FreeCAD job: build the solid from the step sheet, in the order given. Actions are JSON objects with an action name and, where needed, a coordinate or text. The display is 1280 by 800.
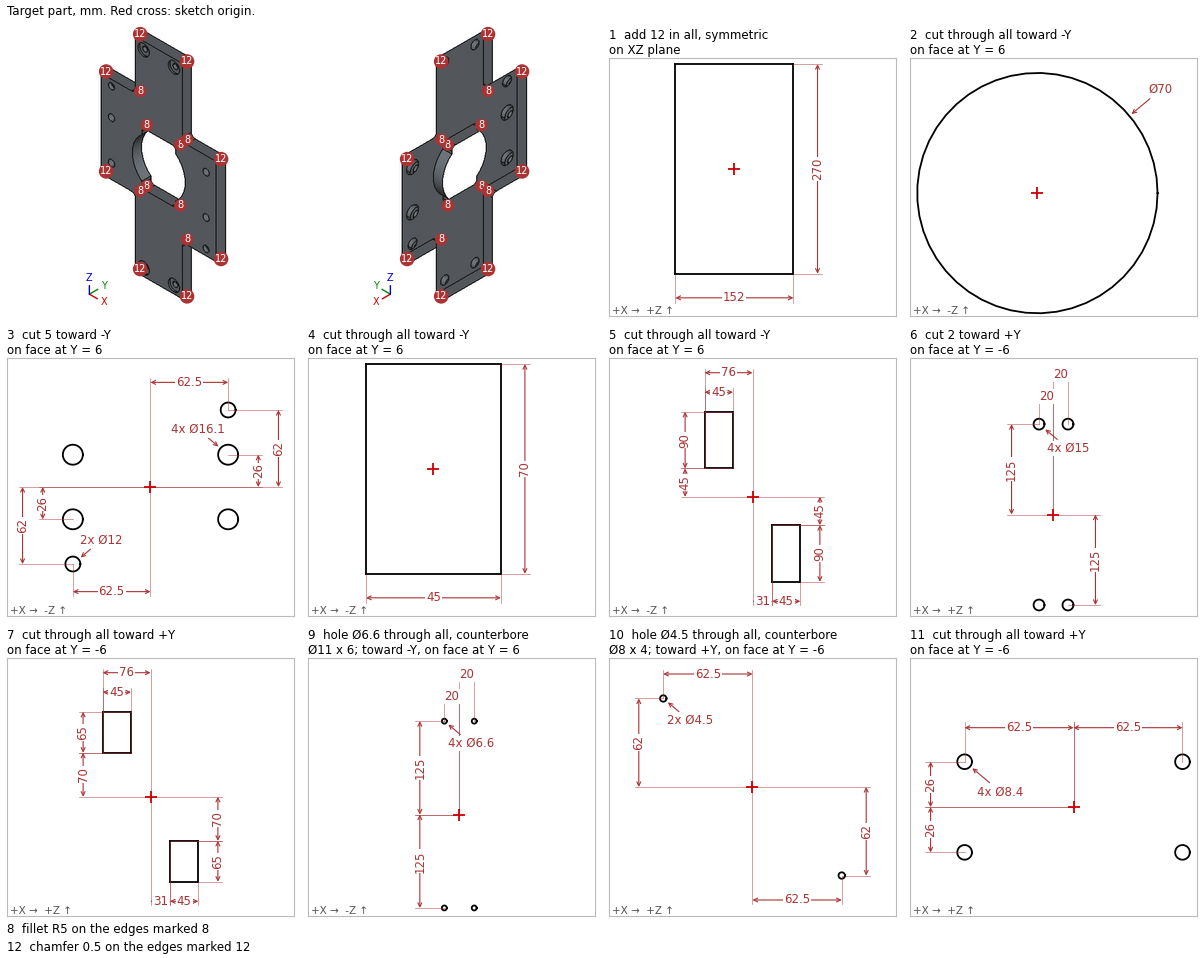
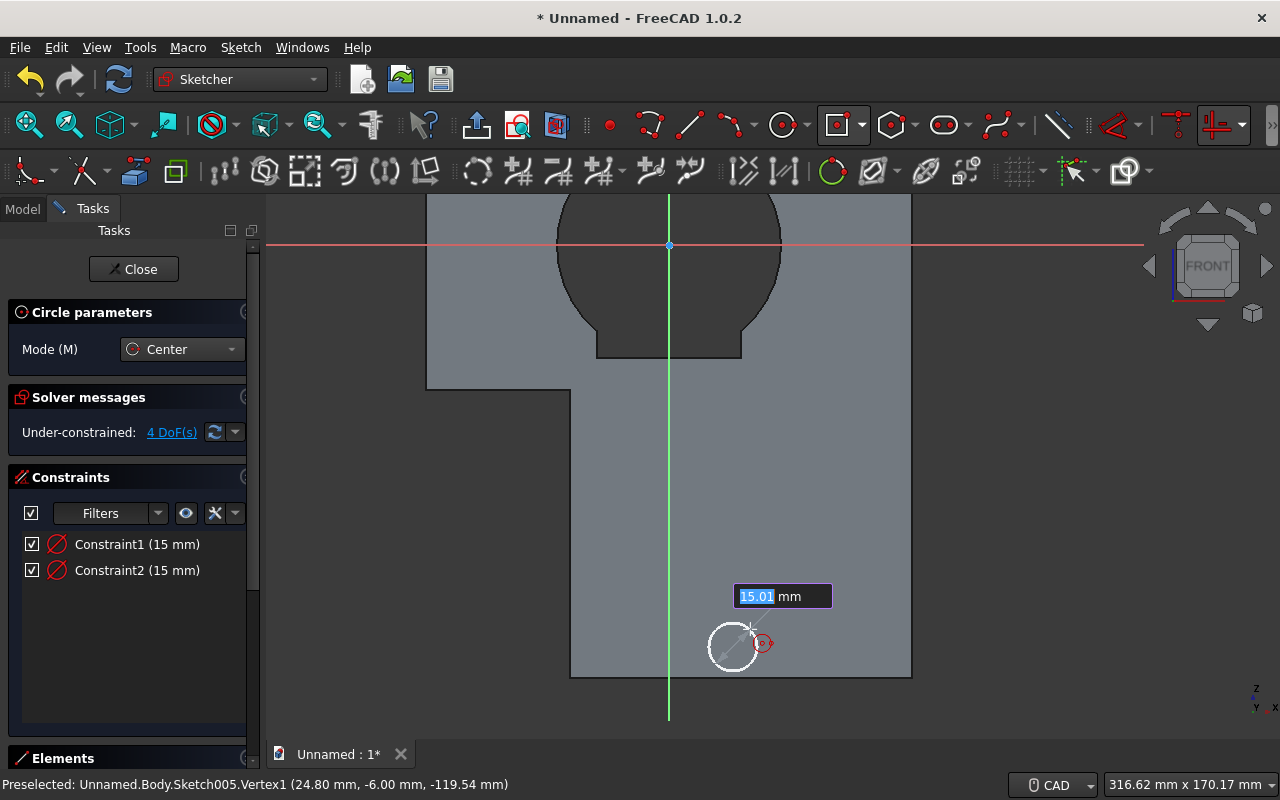
{"action": "type", "text": "15"}
{"action": "key", "text": "Return"}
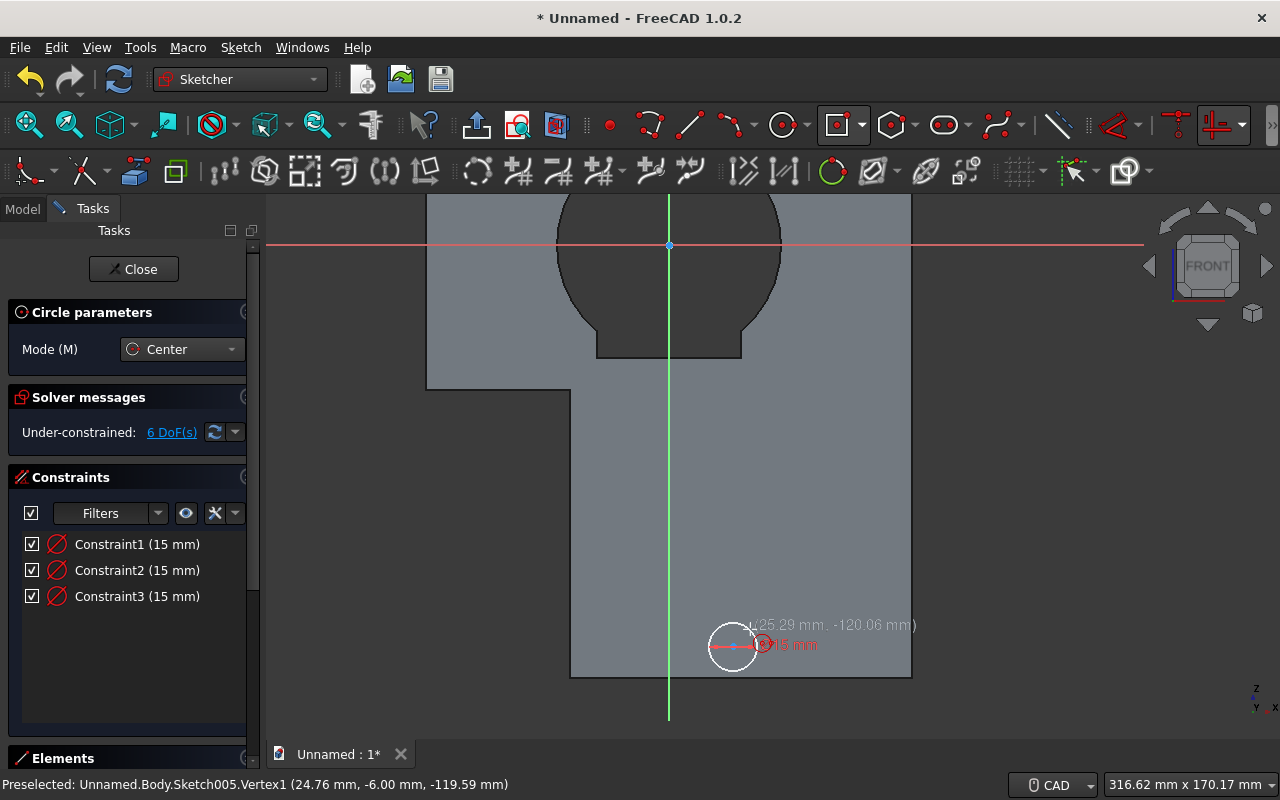
{"action": "left_click", "coordinate": [605, 646]}
{"action": "mouse_move", "coordinate": [622, 629]}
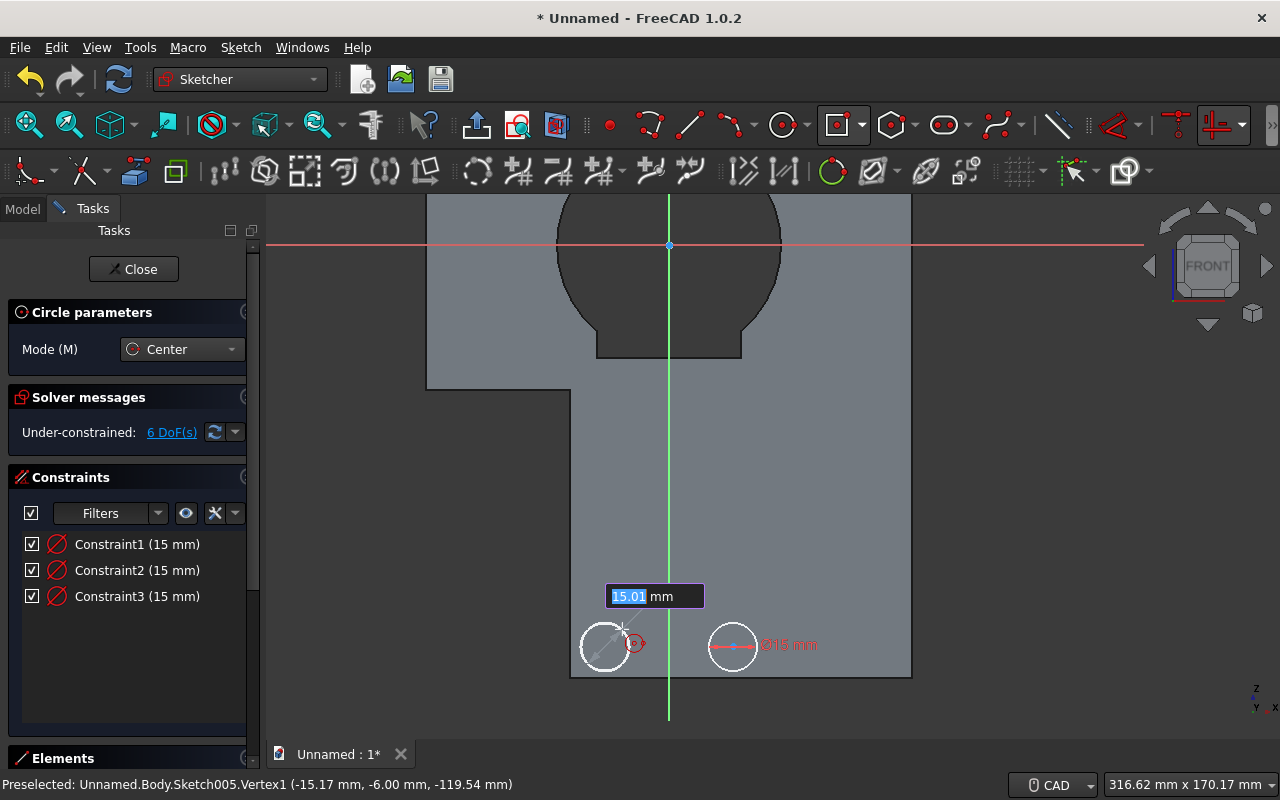
{"action": "type", "text": "15"}
{"action": "key", "text": "Return"}
{"action": "key", "text": "Escape"}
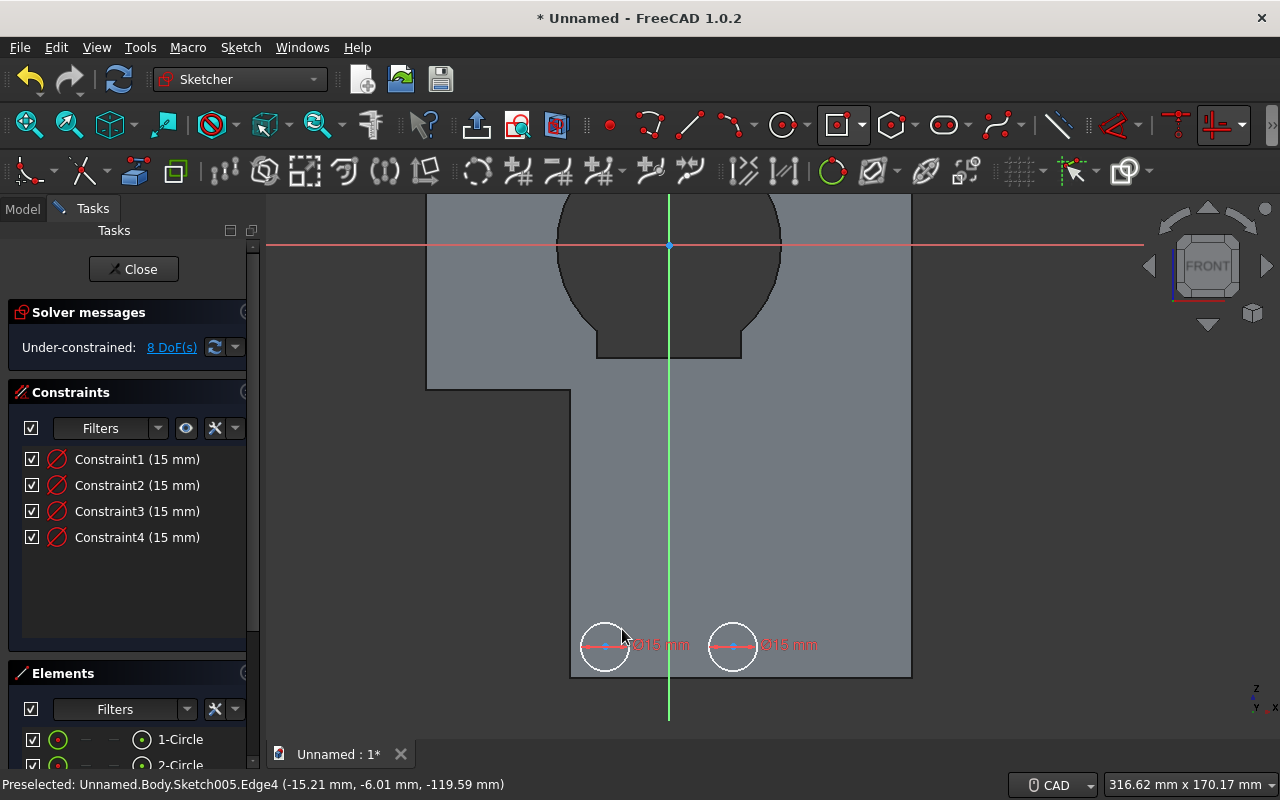
{"action": "scroll", "coordinate": [733, 647], "scroll_direction": "down", "scroll_amount": 4}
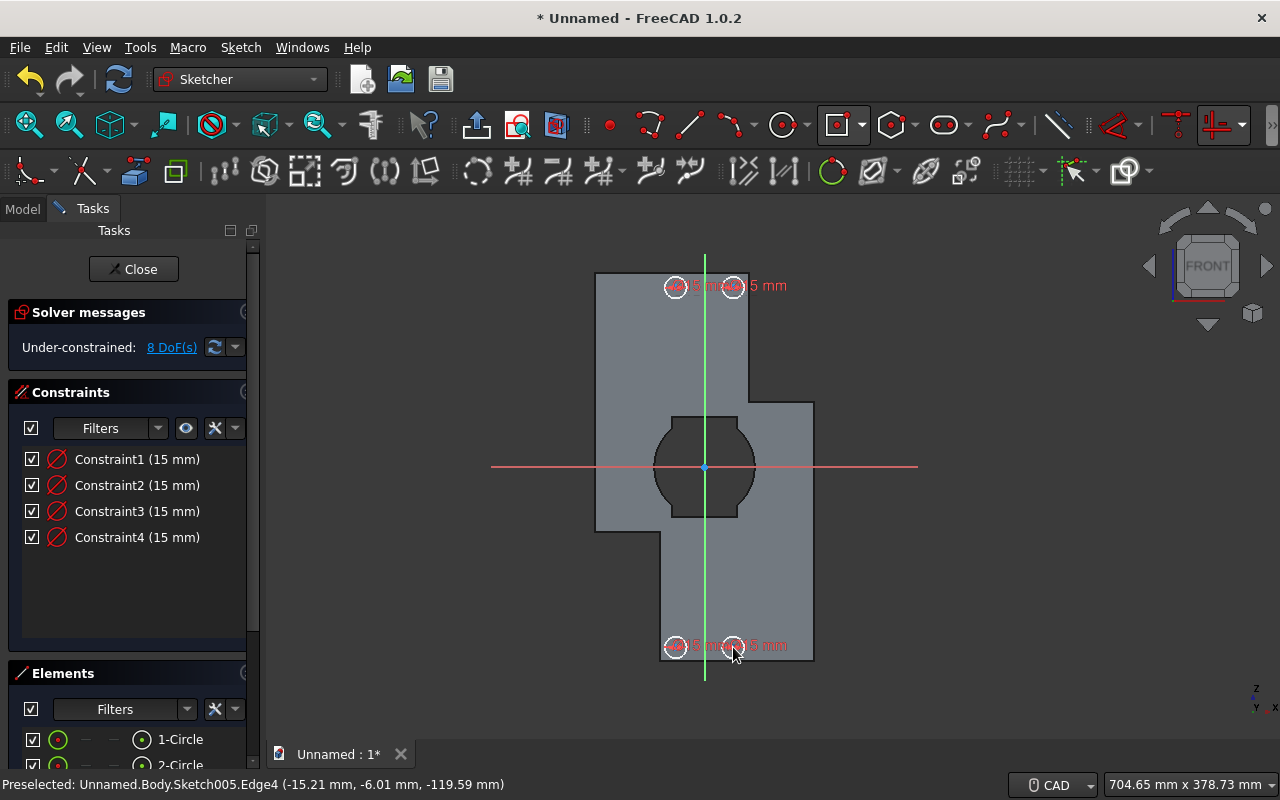
{"action": "left_click", "coordinate": [676, 288]}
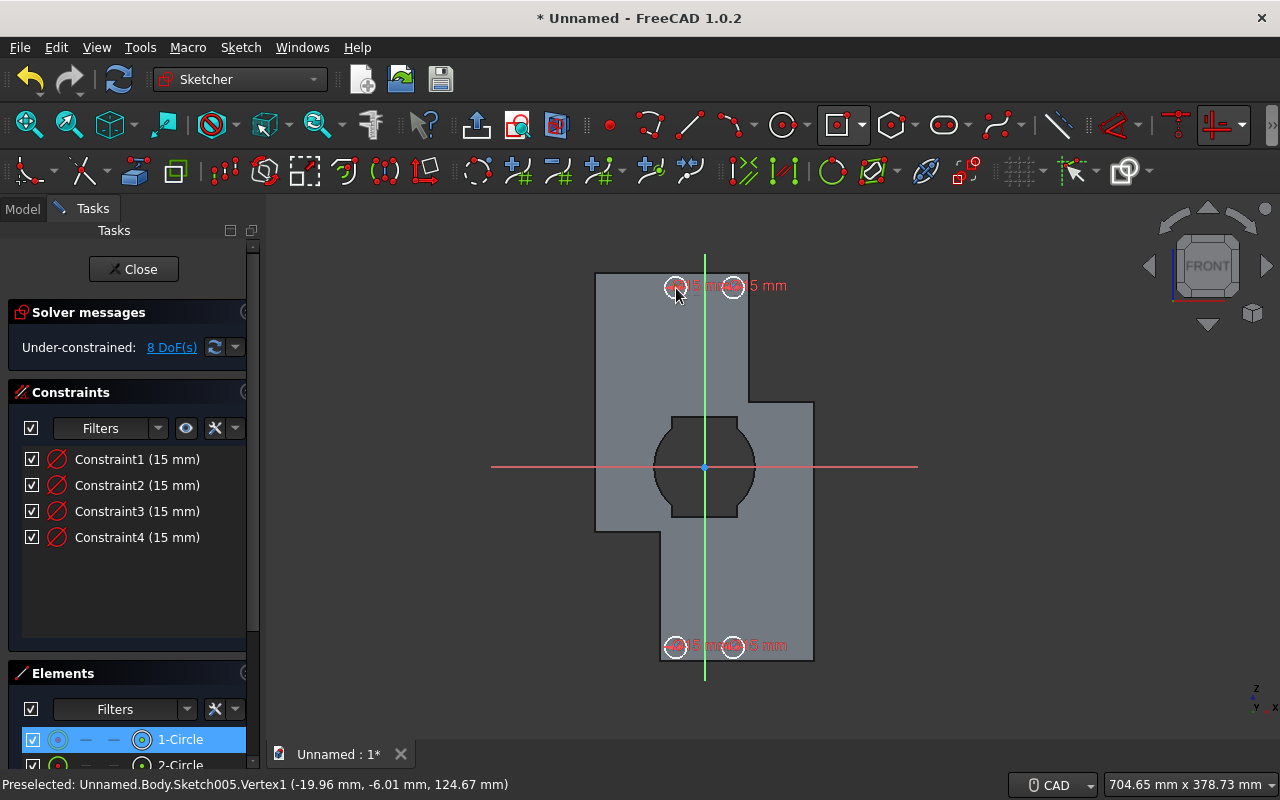
{"action": "left_click", "coordinate": [733, 288]}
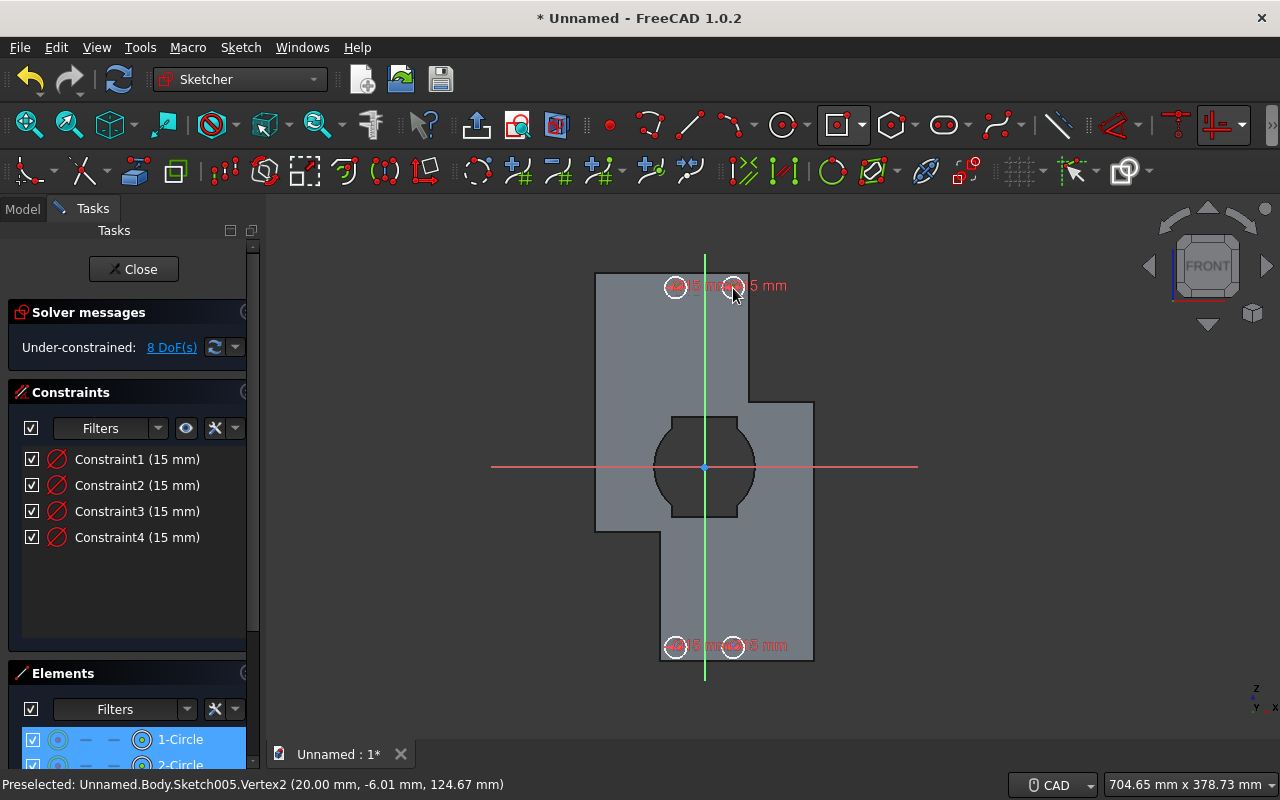
{"action": "key", "text": "h"}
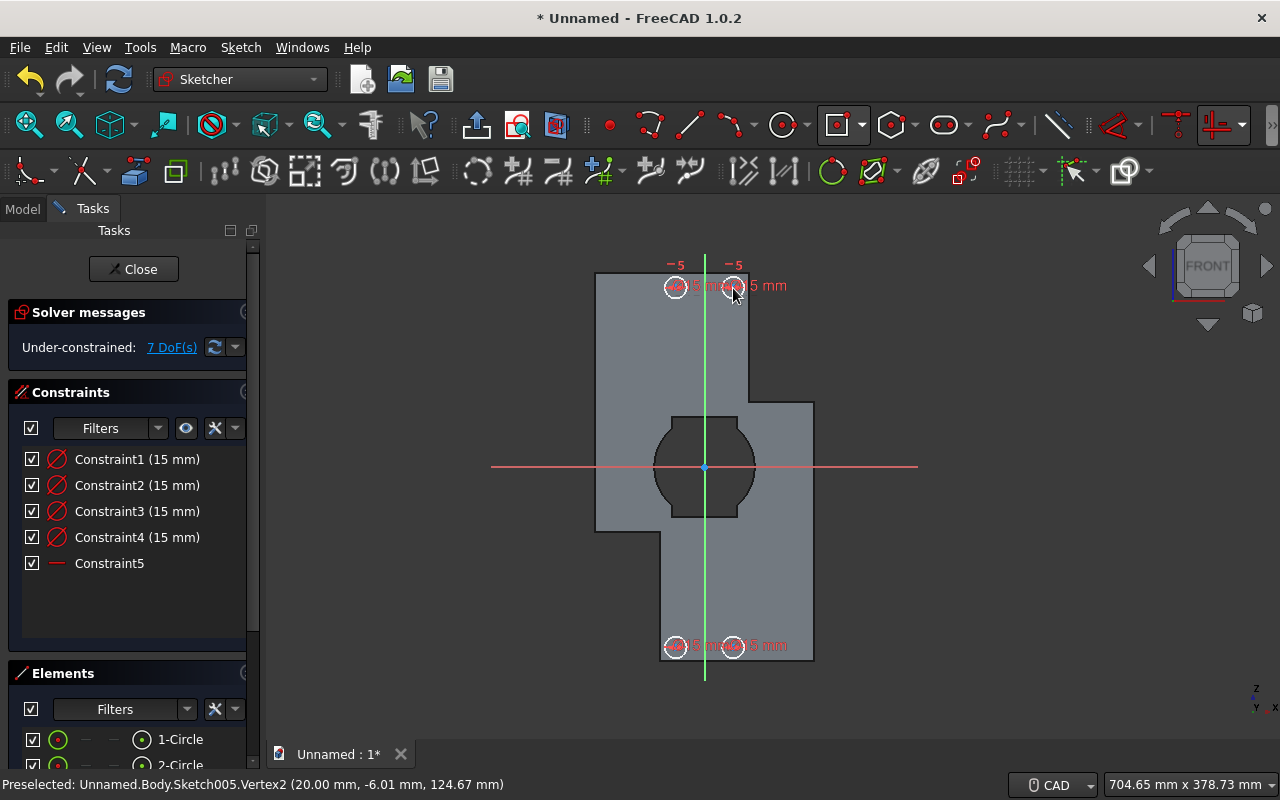
{"action": "left_click", "coordinate": [733, 288]}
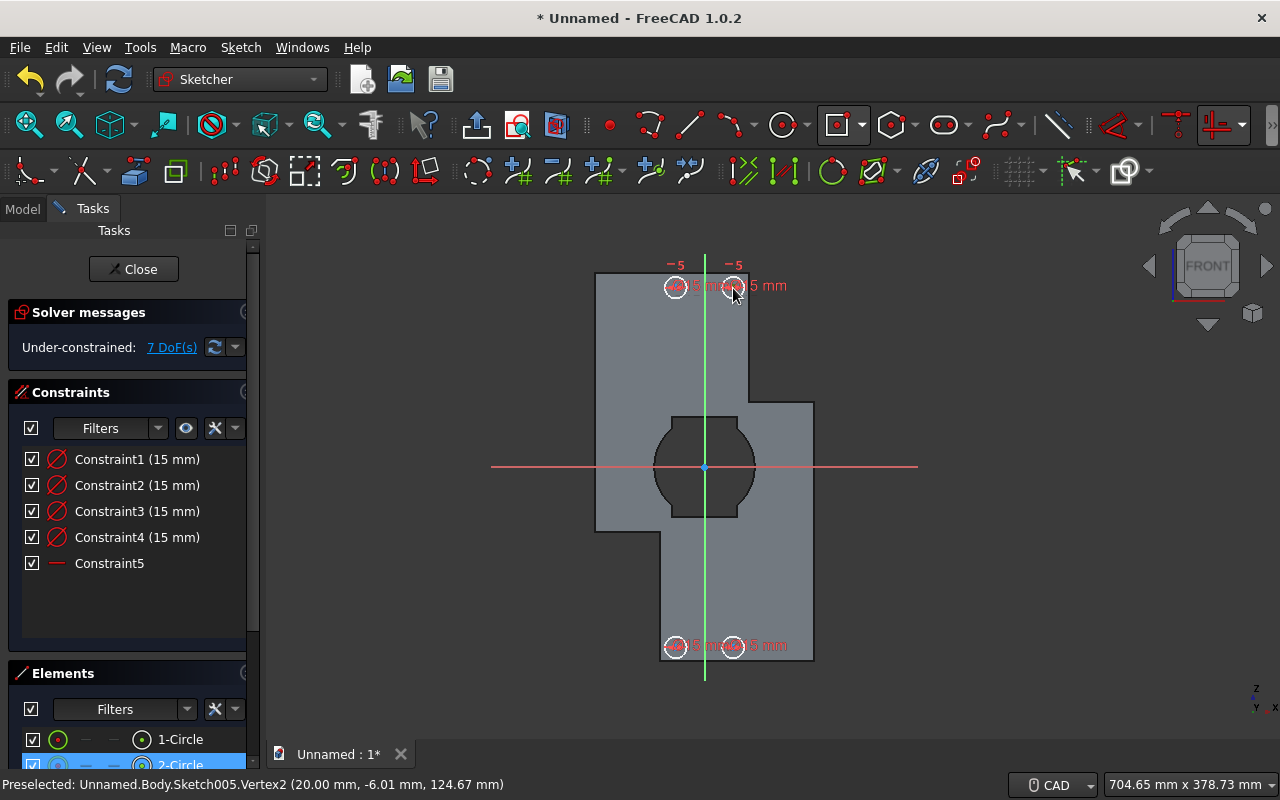
{"action": "left_click", "coordinate": [733, 647]}